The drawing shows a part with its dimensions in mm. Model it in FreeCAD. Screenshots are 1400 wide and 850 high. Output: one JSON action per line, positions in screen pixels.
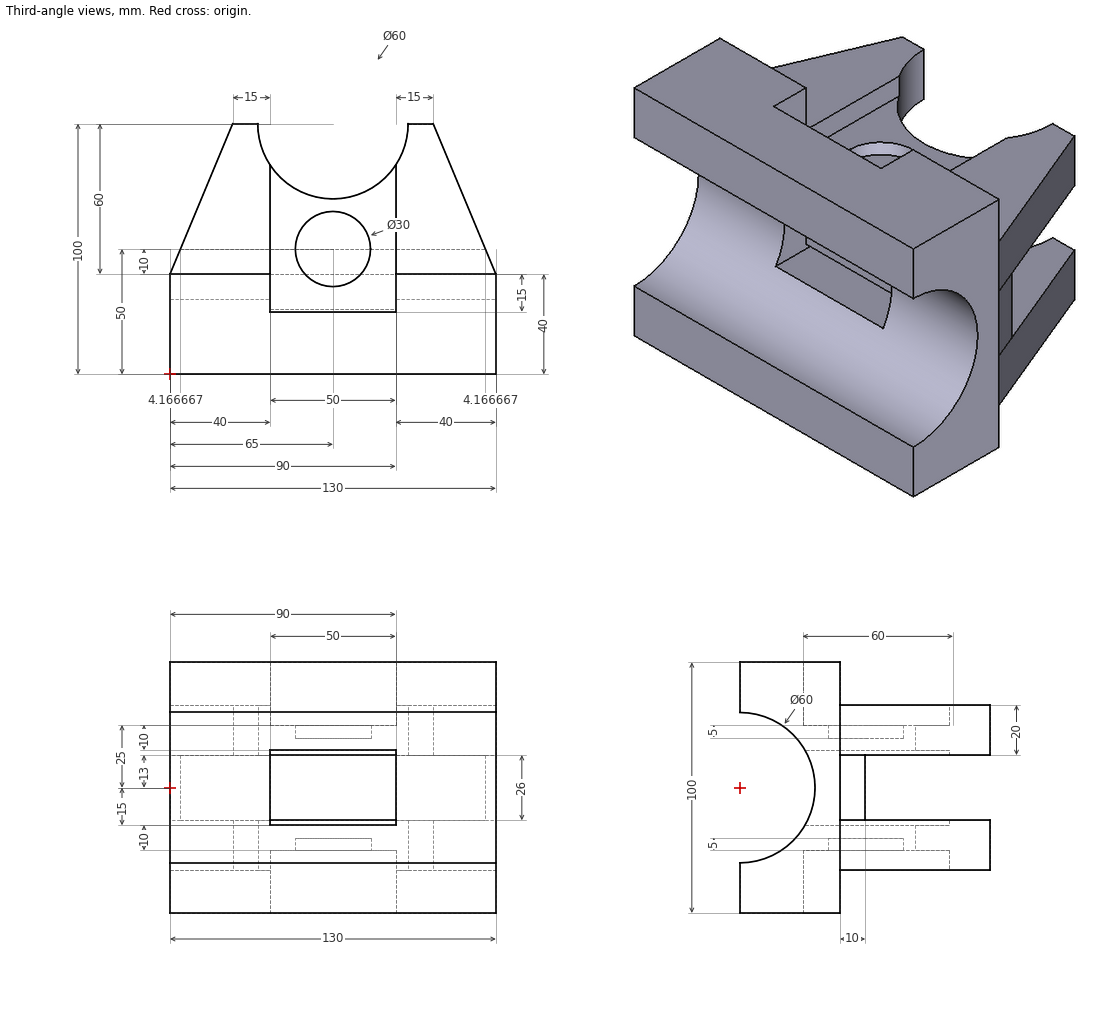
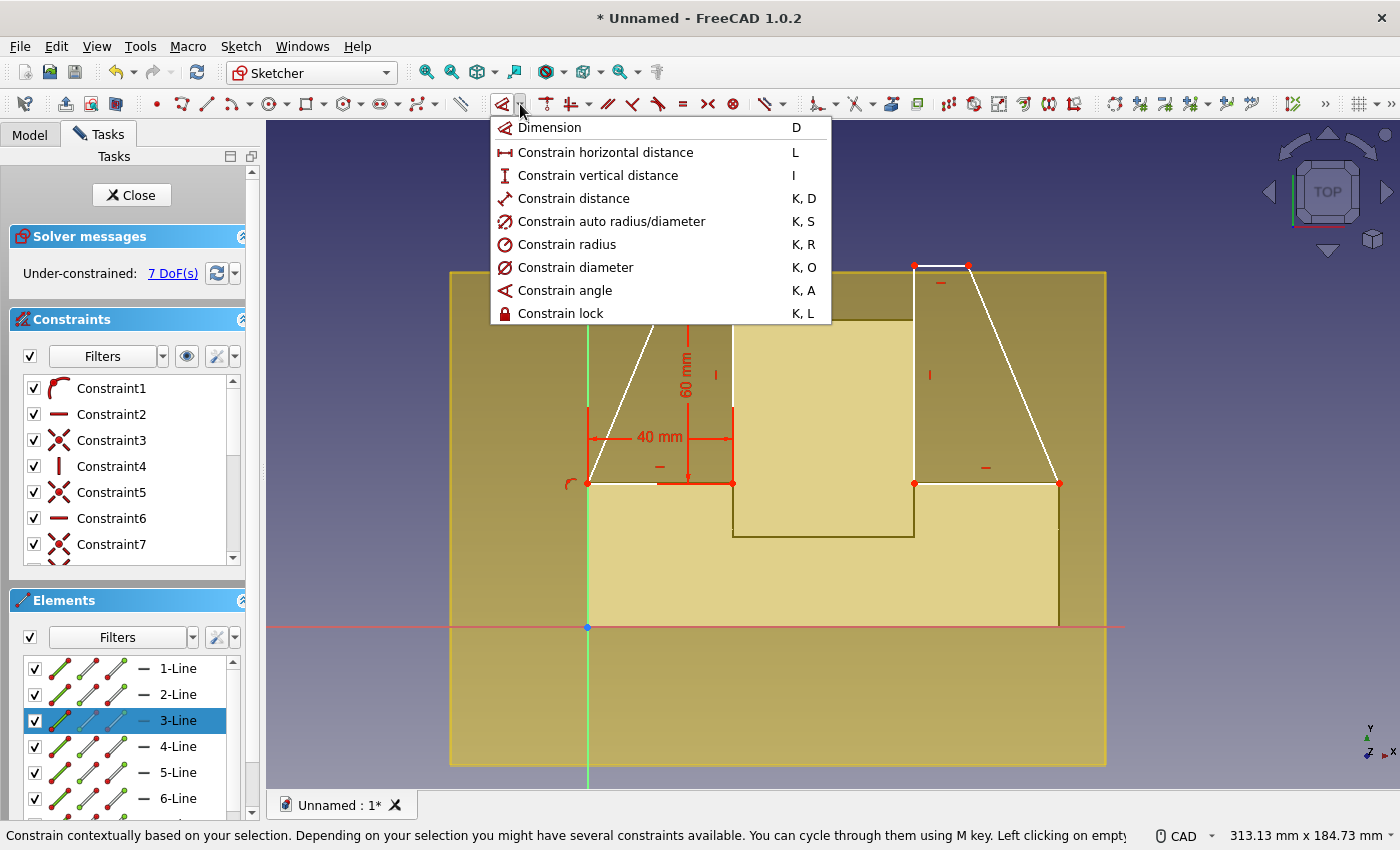
{"action": "left_click", "coordinate": [661, 152]}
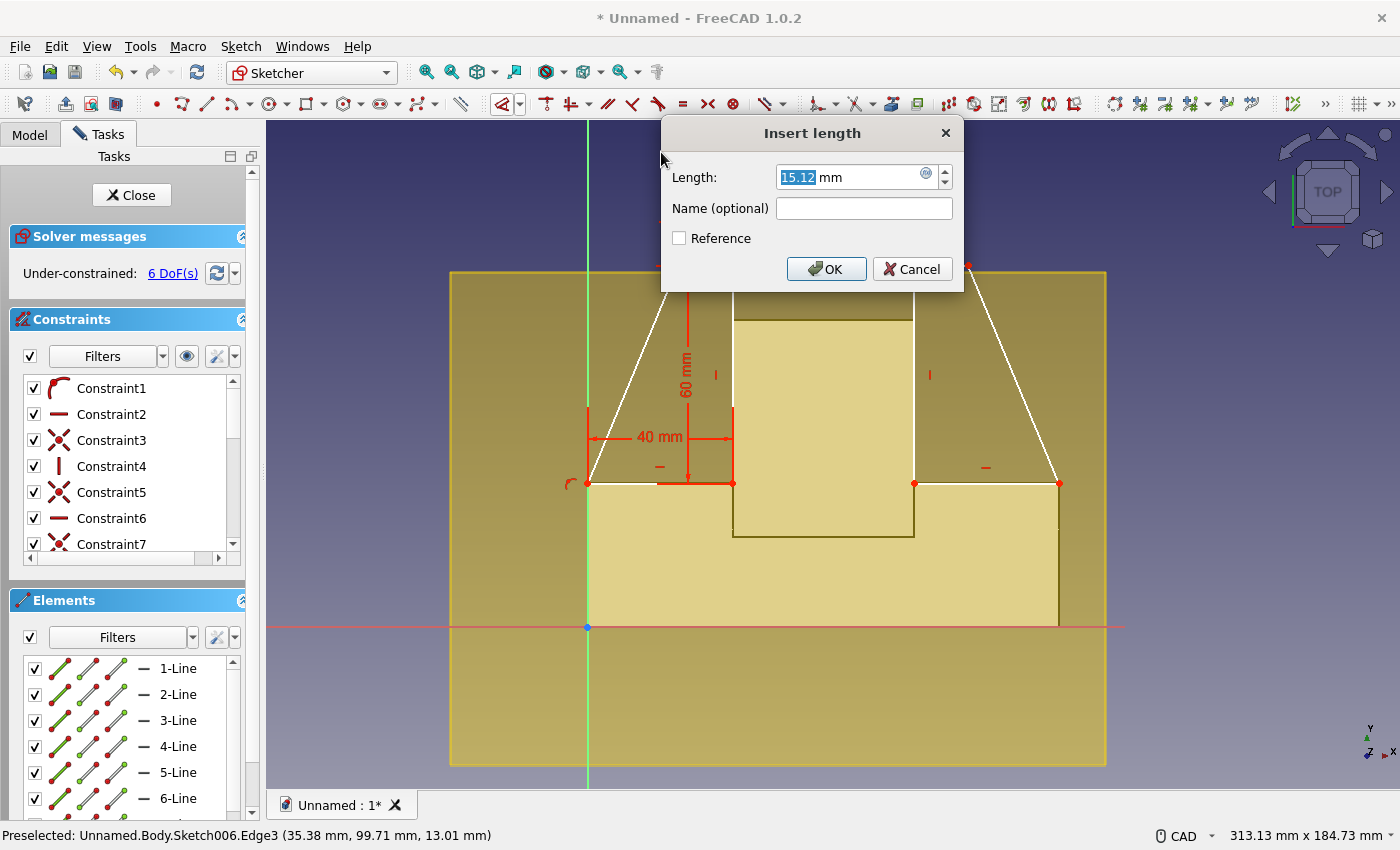
{"action": "type", "text": "15"}
{"action": "key", "text": "Return"}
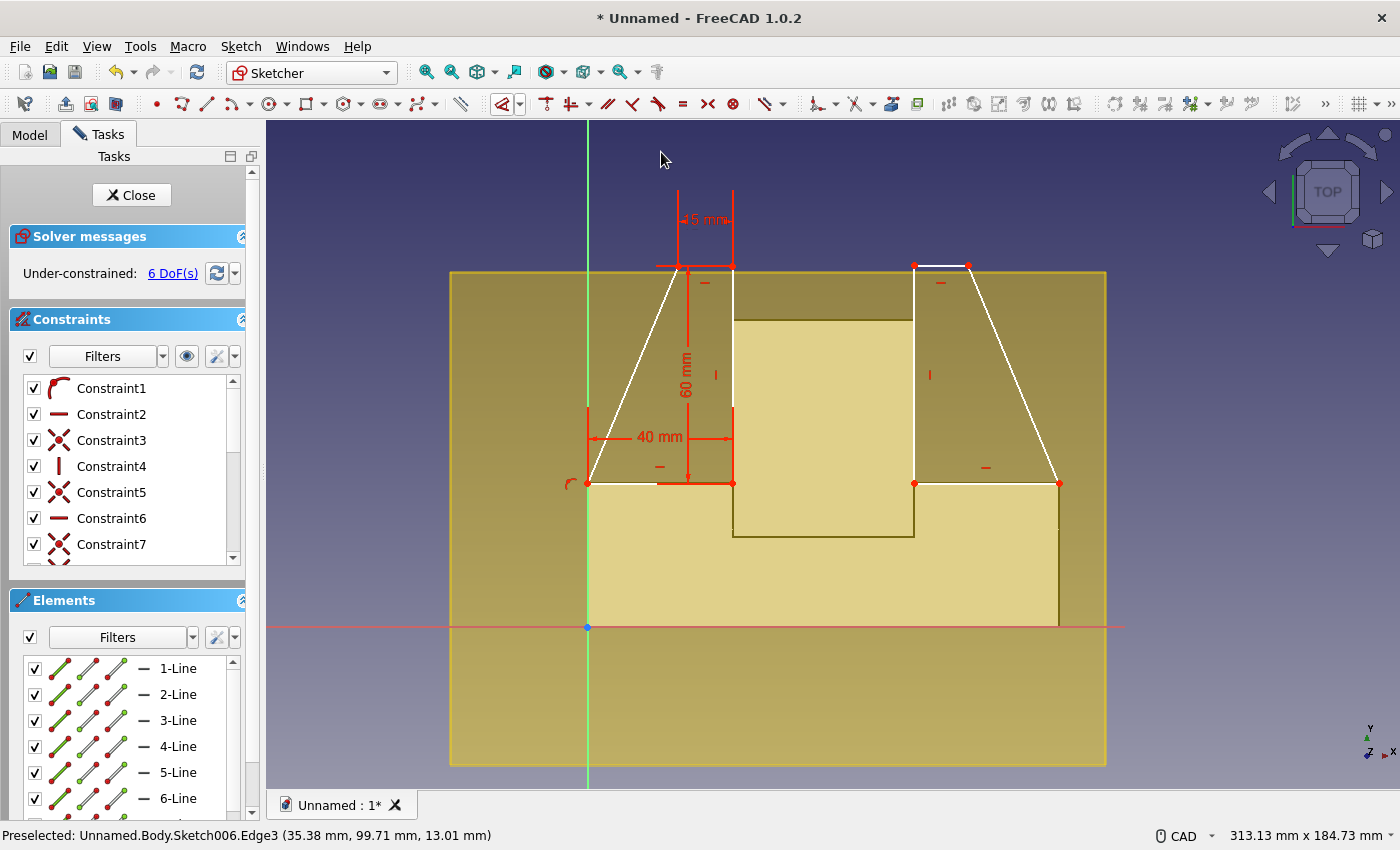
{"action": "left_click", "coordinate": [958, 484]}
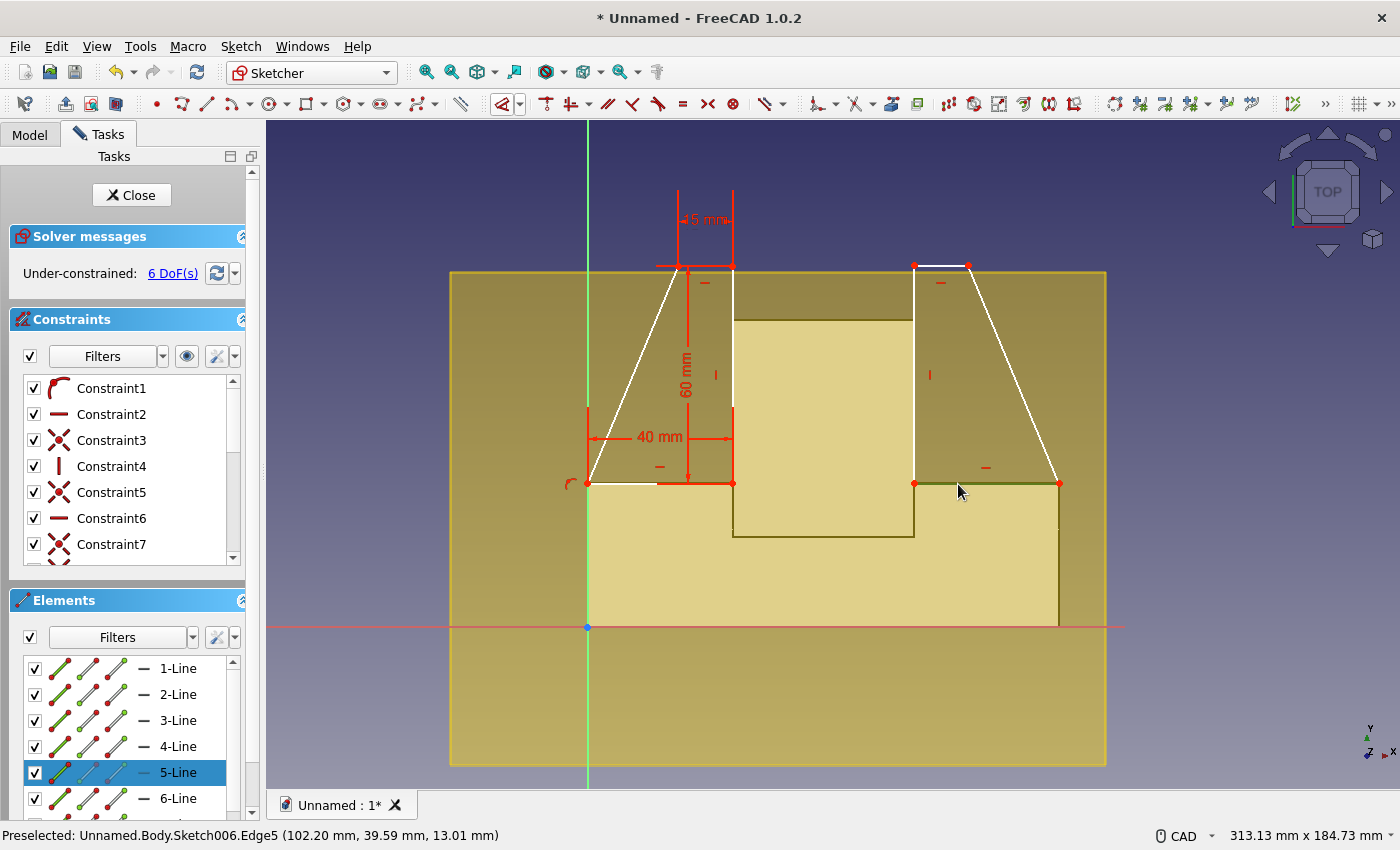
{"action": "key", "text": "l"}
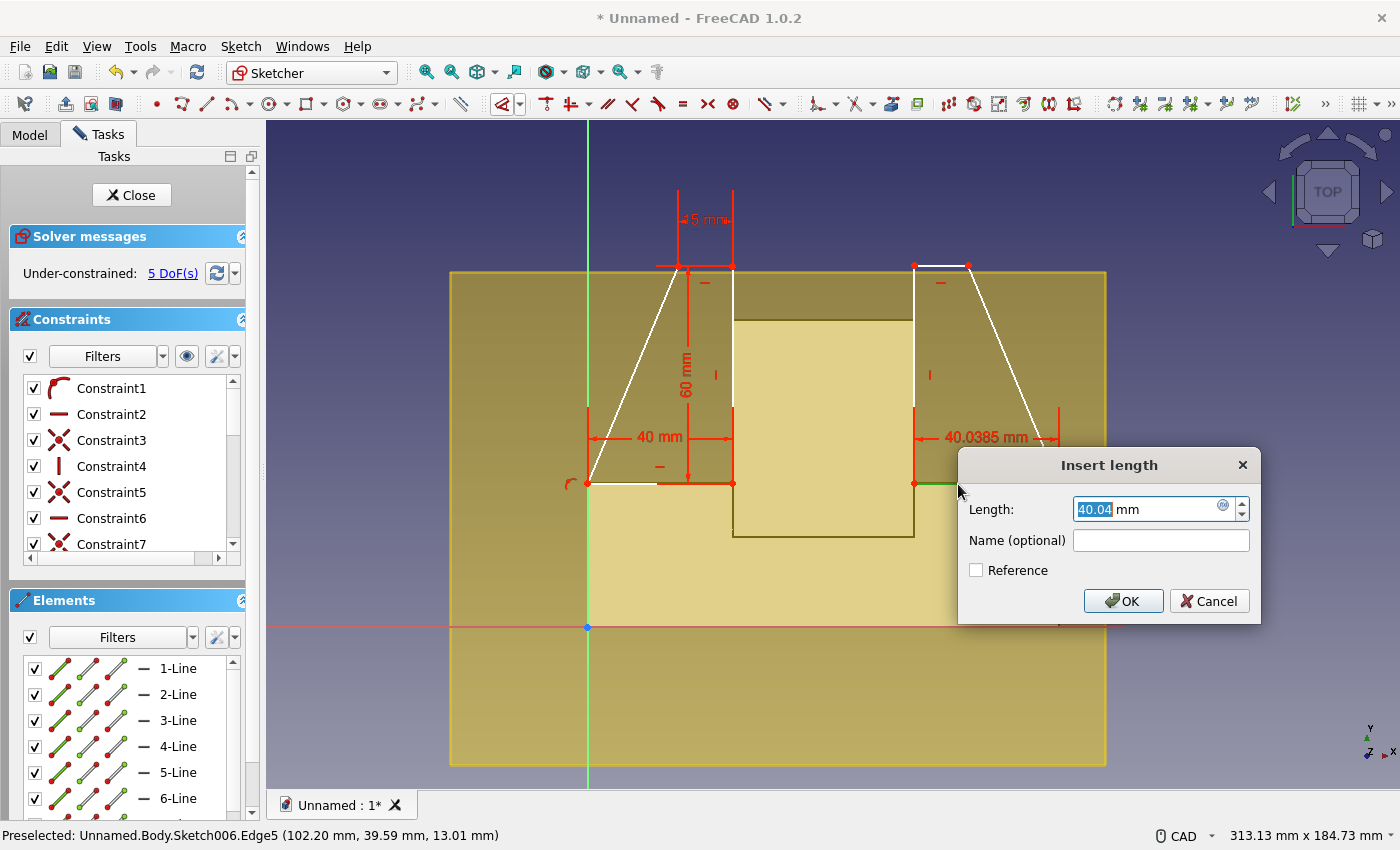
{"action": "type", "text": "40"}
{"action": "key", "text": "Return"}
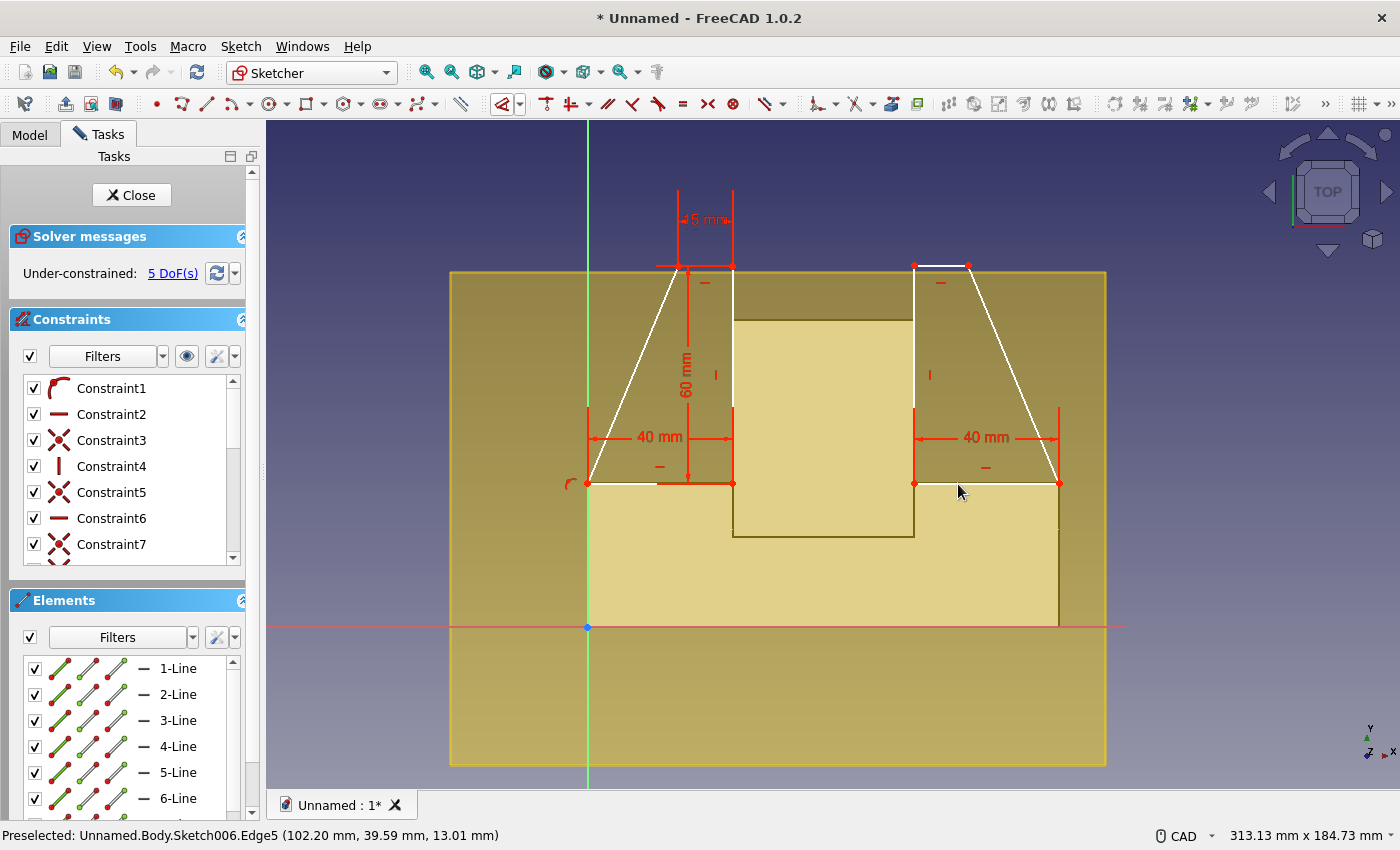
{"action": "left_click", "coordinate": [952, 266]}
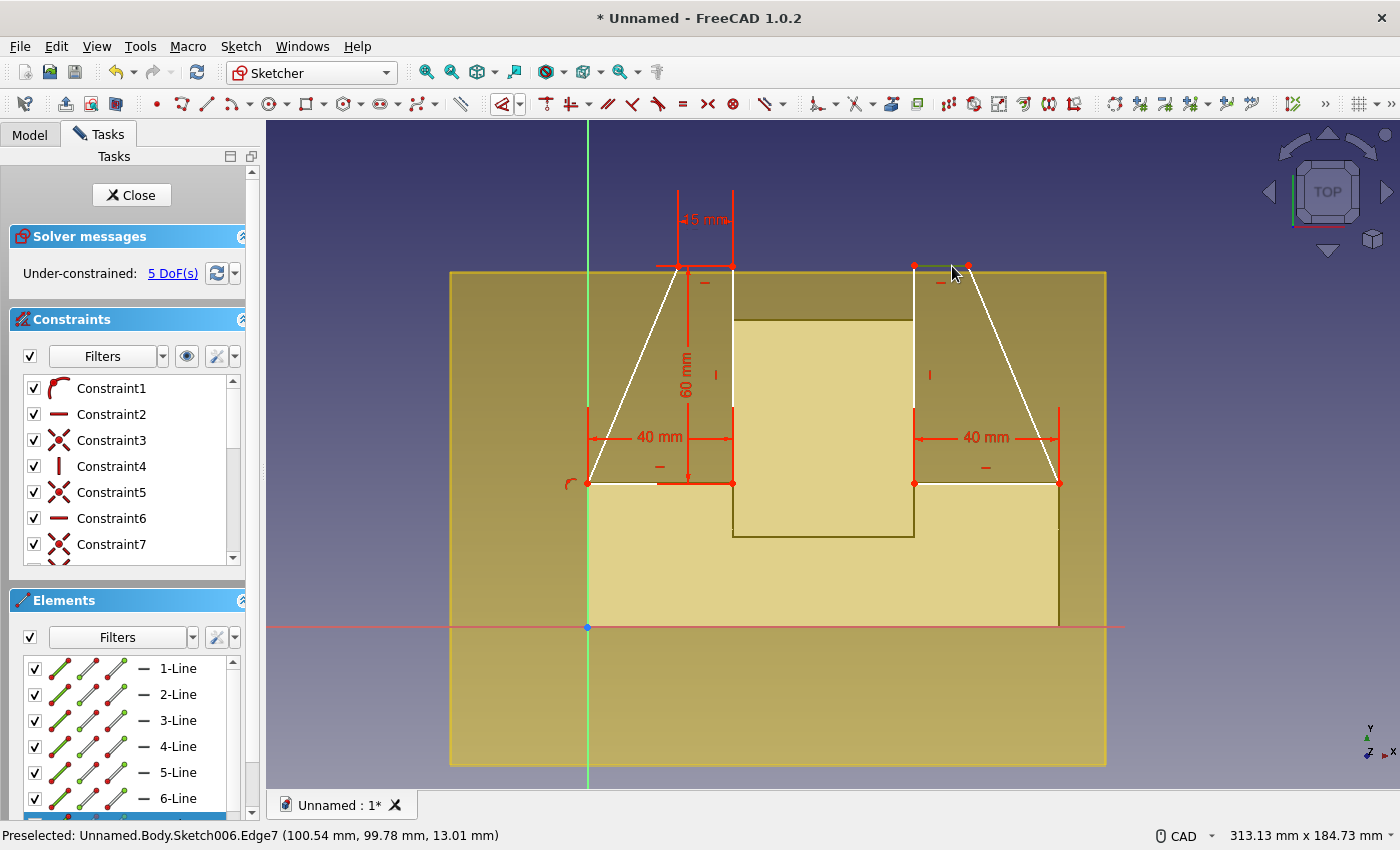
{"action": "key", "text": "l"}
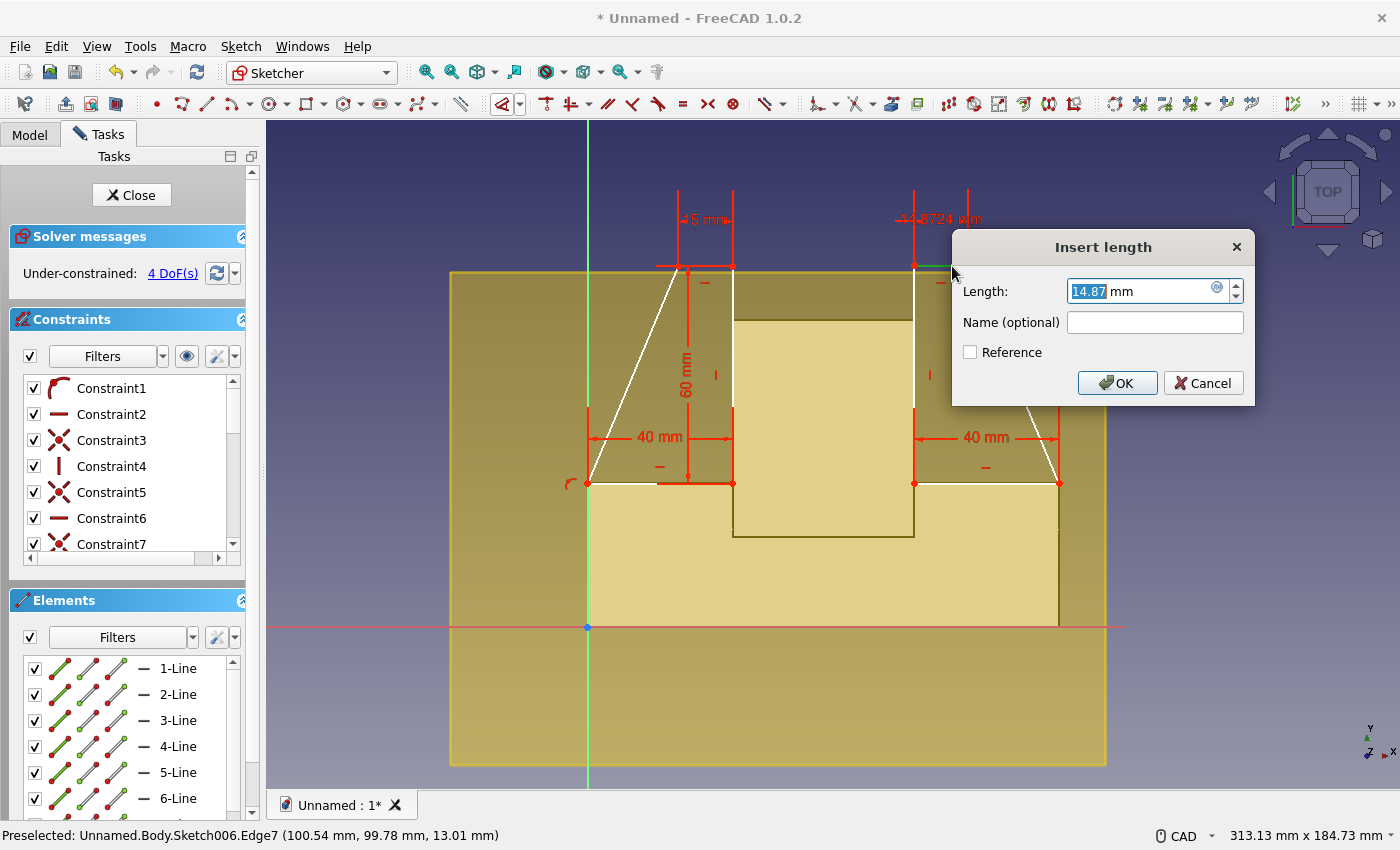
{"action": "type", "text": "15"}
{"action": "key", "text": "Return"}